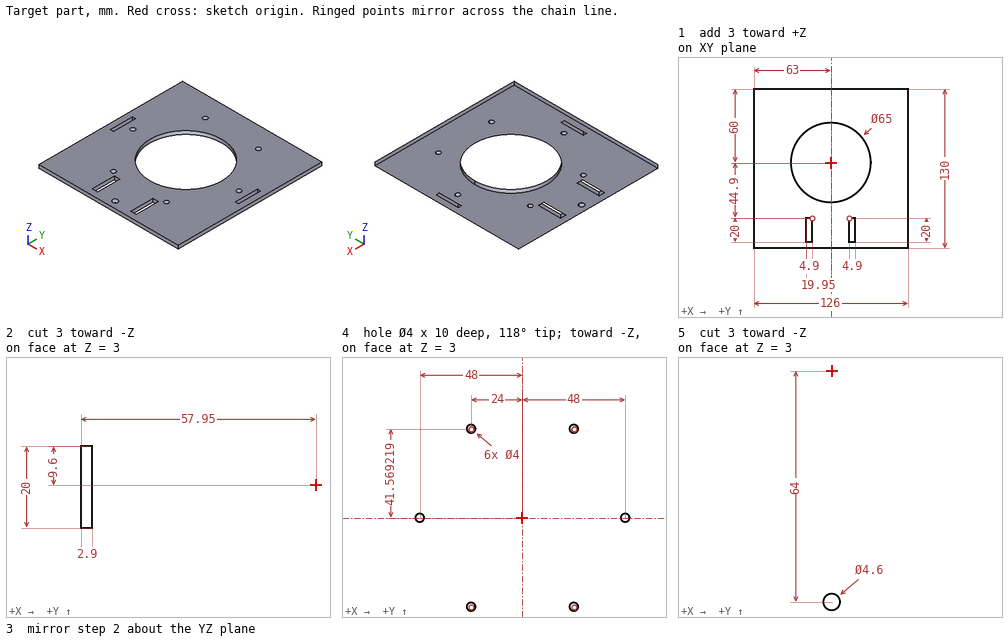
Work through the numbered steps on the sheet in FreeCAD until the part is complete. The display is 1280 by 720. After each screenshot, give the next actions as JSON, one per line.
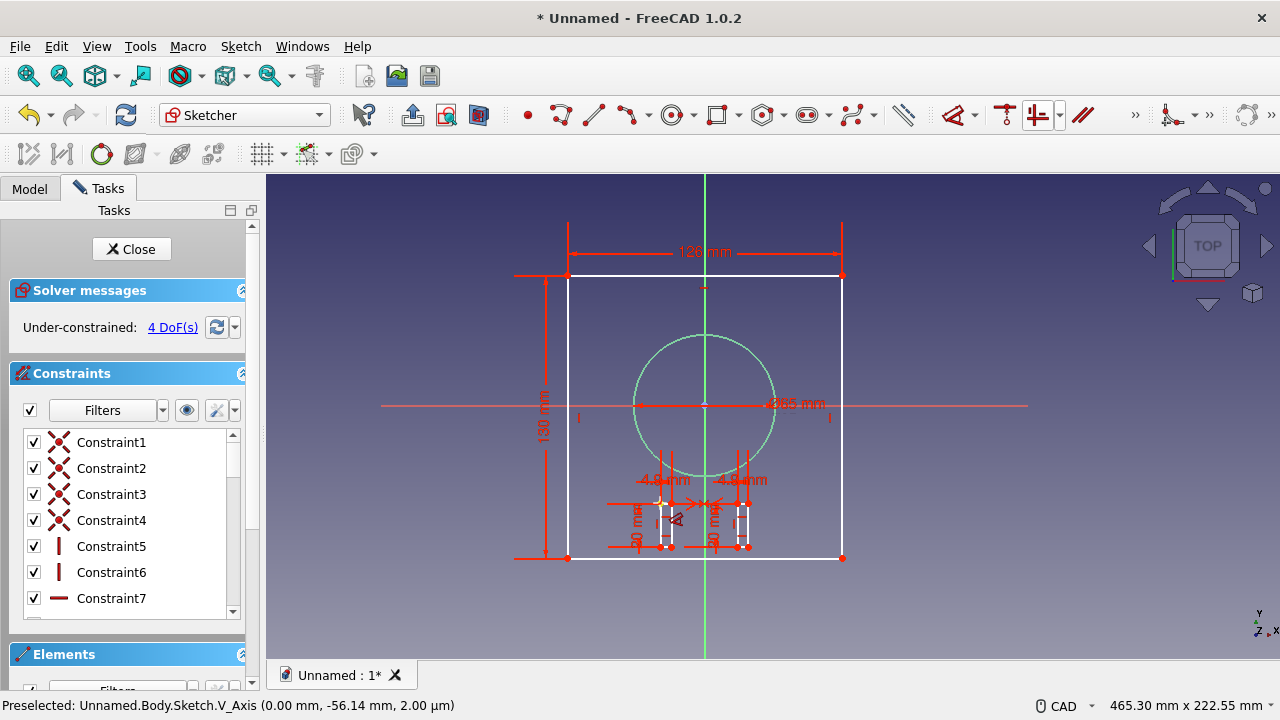
{"action": "left_click", "coordinate": [568, 276]}
{"action": "left_click", "coordinate": [636, 242]}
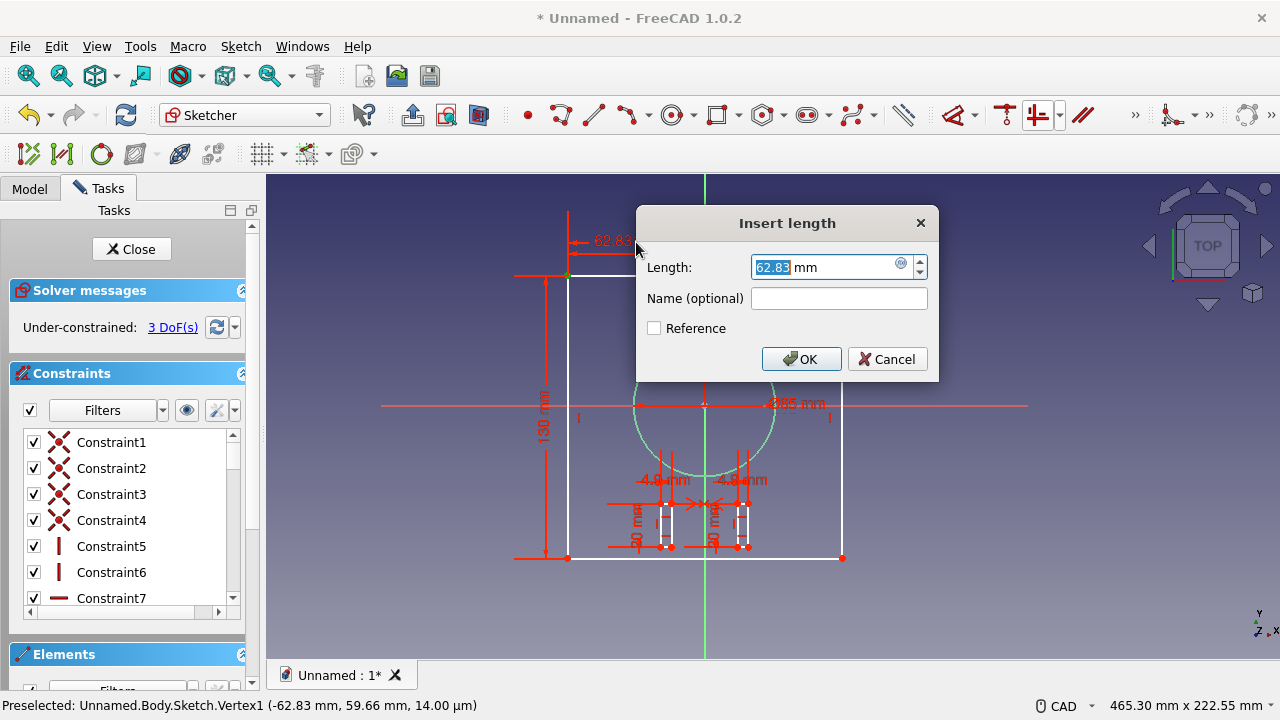
{"action": "type", "text": "63"}
{"action": "key", "text": "Return"}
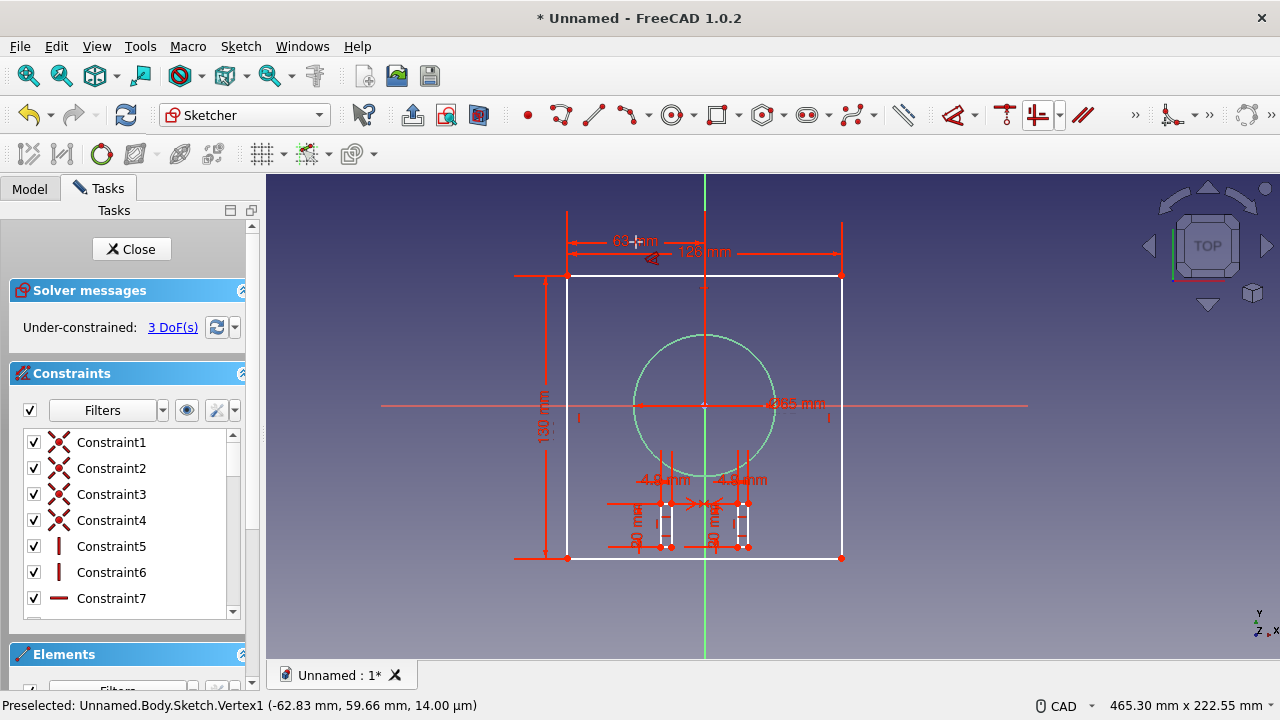
{"action": "left_click", "coordinate": [567, 276]}
{"action": "left_click", "coordinate": [533, 341]}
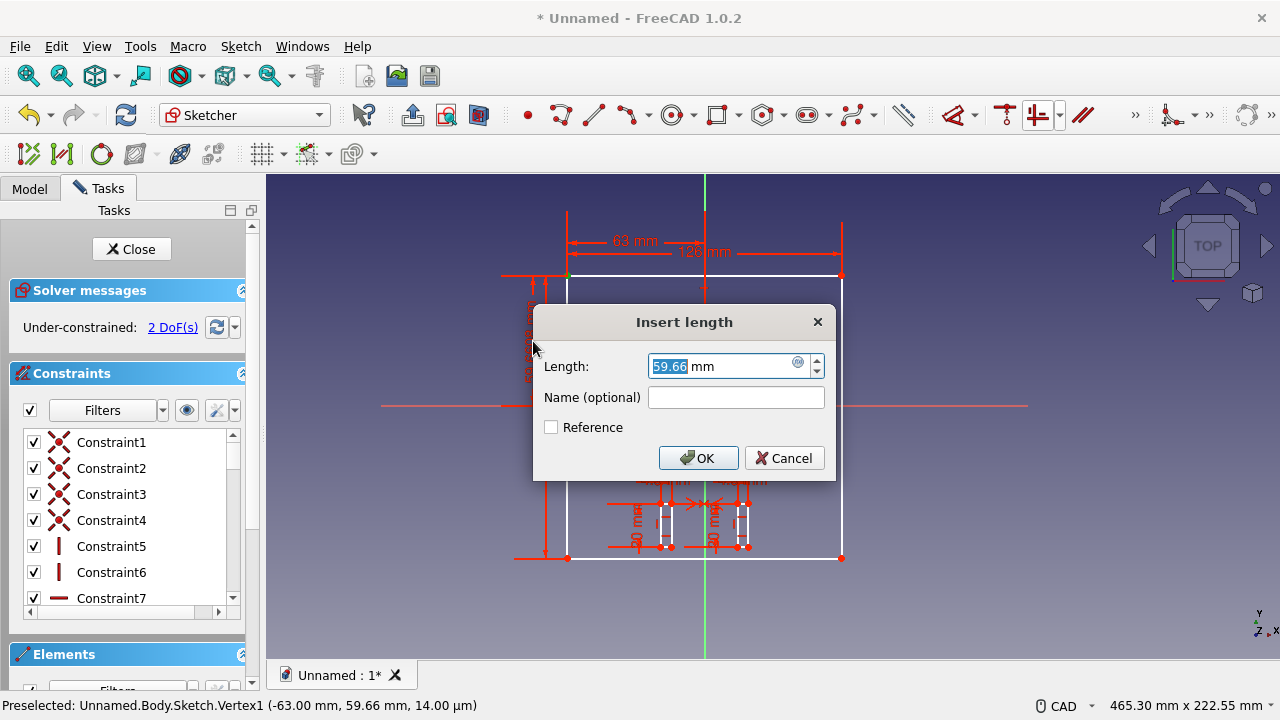
{"action": "type", "text": "60"}
{"action": "key", "text": "Return"}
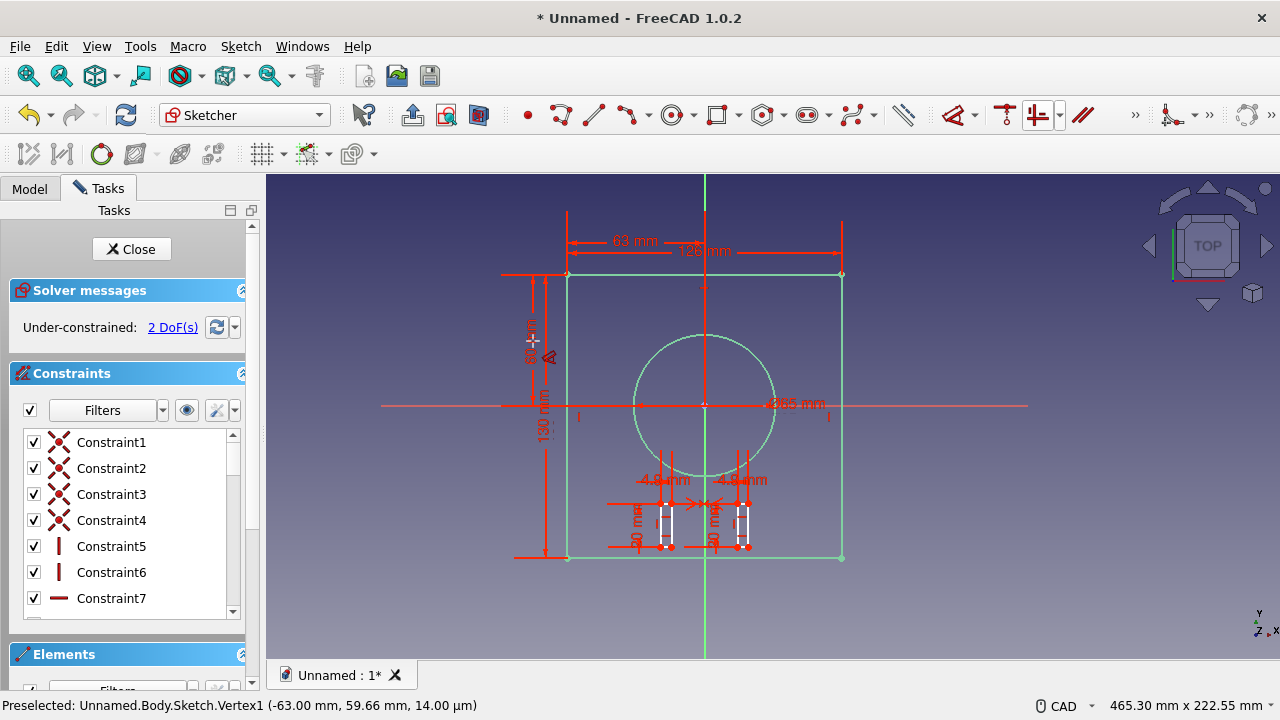
{"action": "left_click", "coordinate": [661, 504]}
{"action": "left_click", "coordinate": [627, 455]}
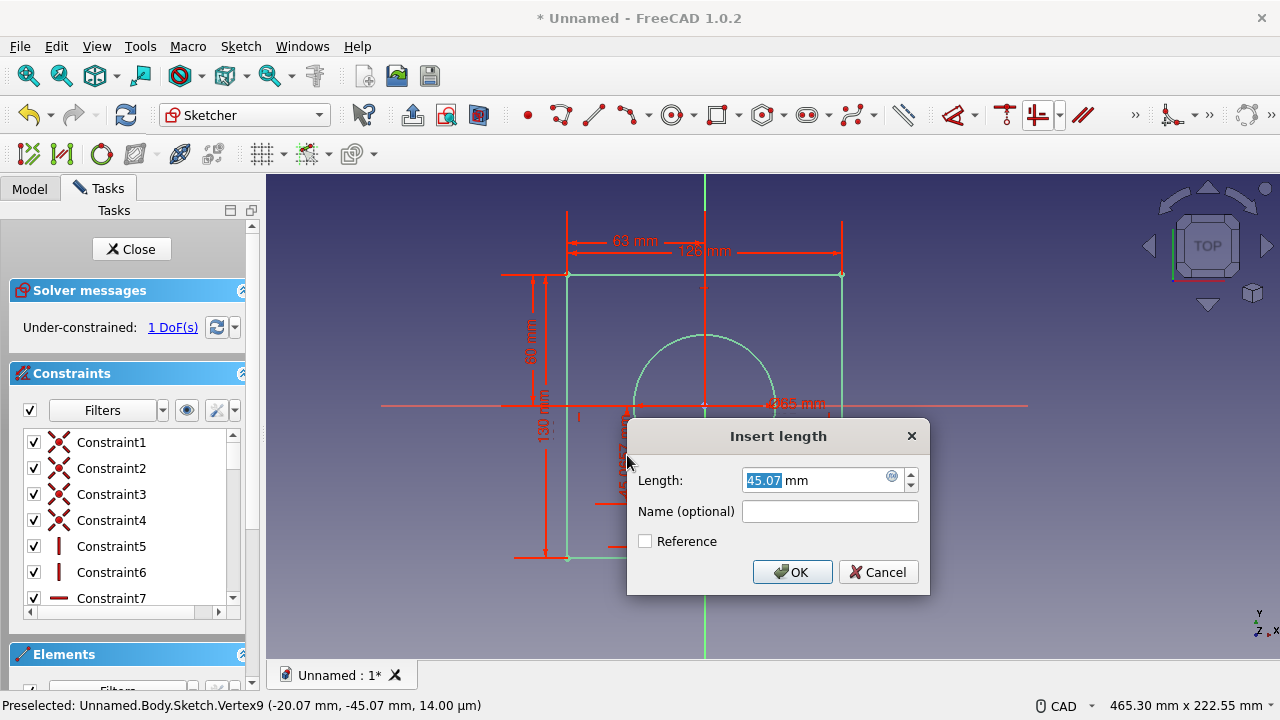
{"action": "type", "text": "44.9"}
{"action": "key", "text": "Return"}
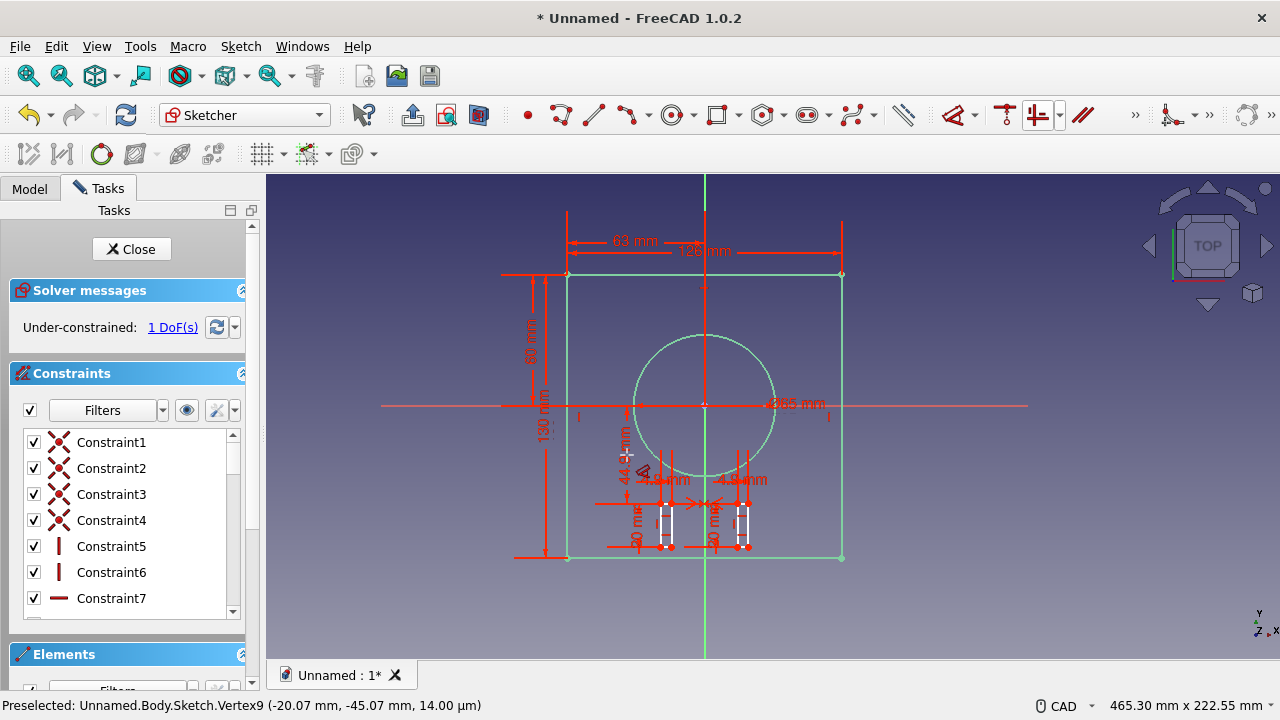
{"action": "left_click", "coordinate": [661, 504]}
{"action": "left_click", "coordinate": [683, 372]}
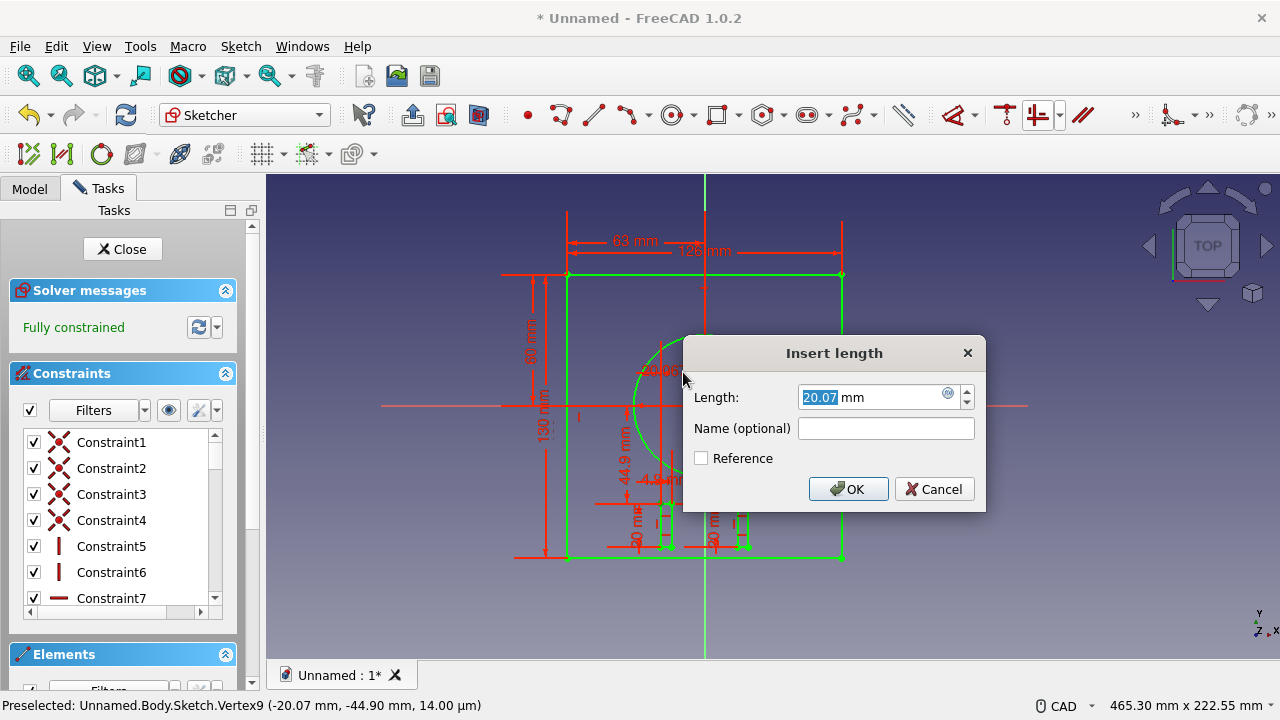
{"action": "type", "text": "19.95"}
{"action": "key", "text": "Return"}
{"action": "key", "text": "Escape"}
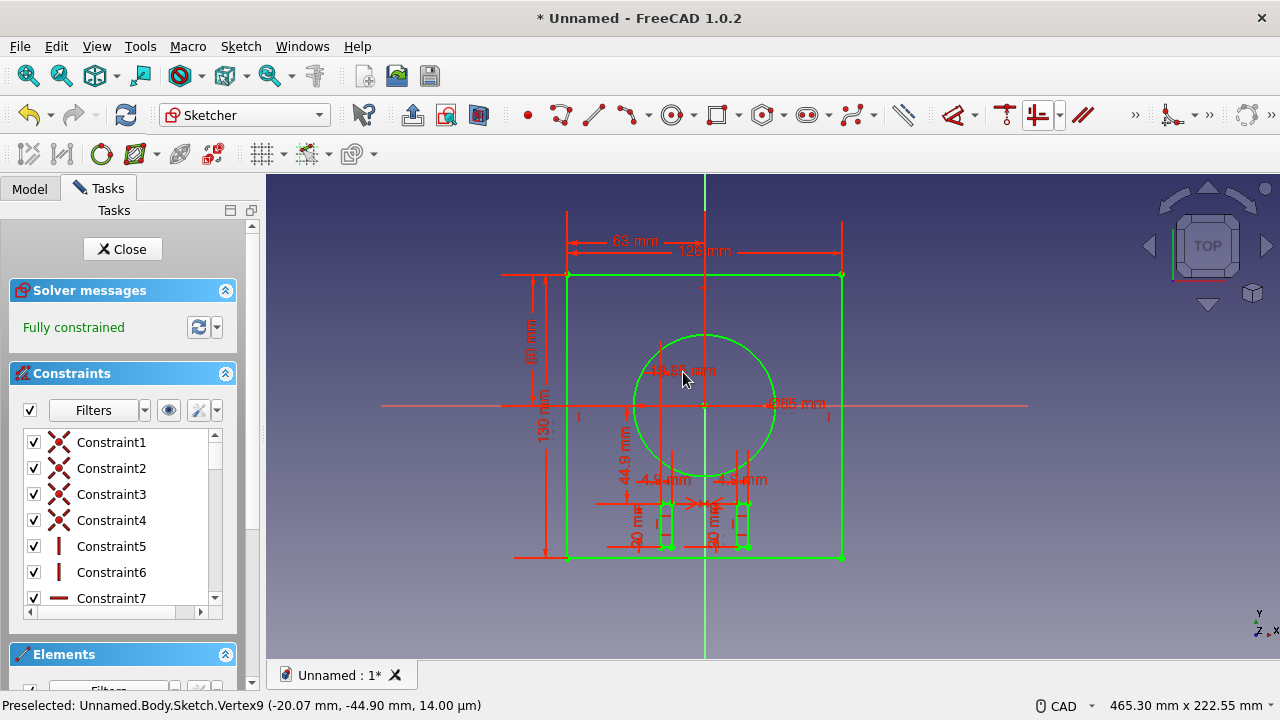
{"action": "left_click", "coordinate": [123, 249]}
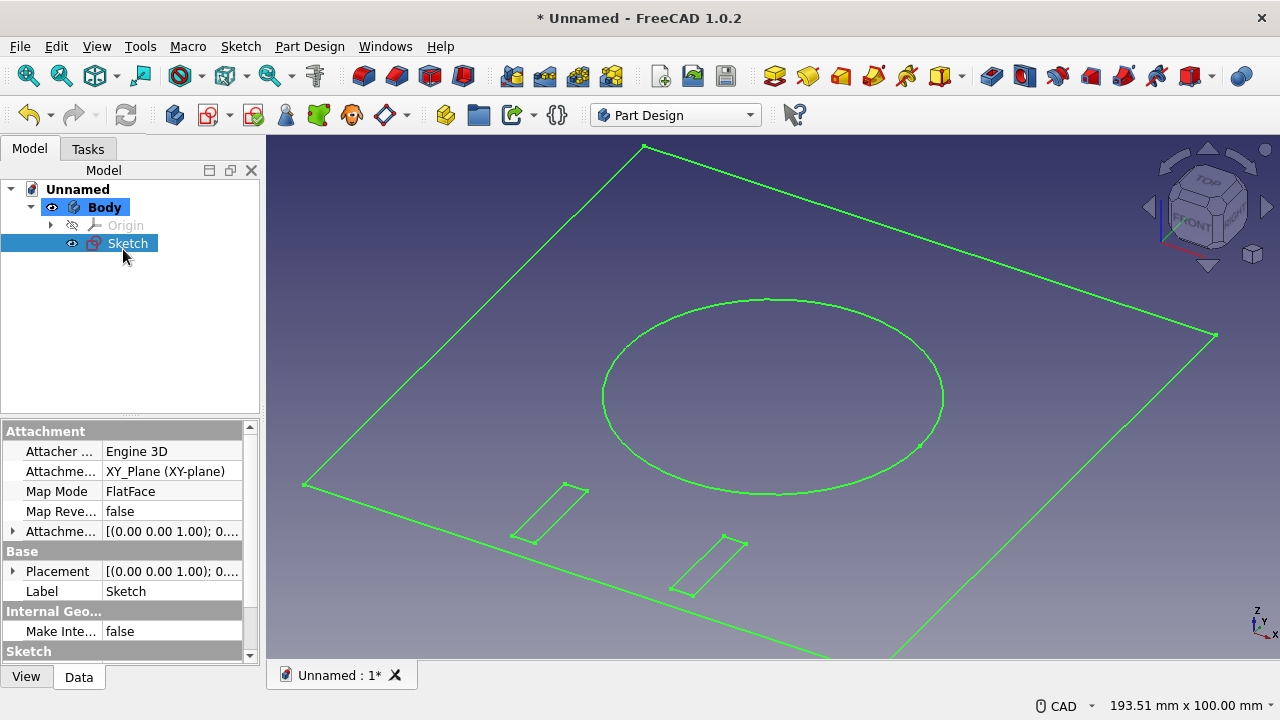
{"action": "left_click", "coordinate": [775, 76]}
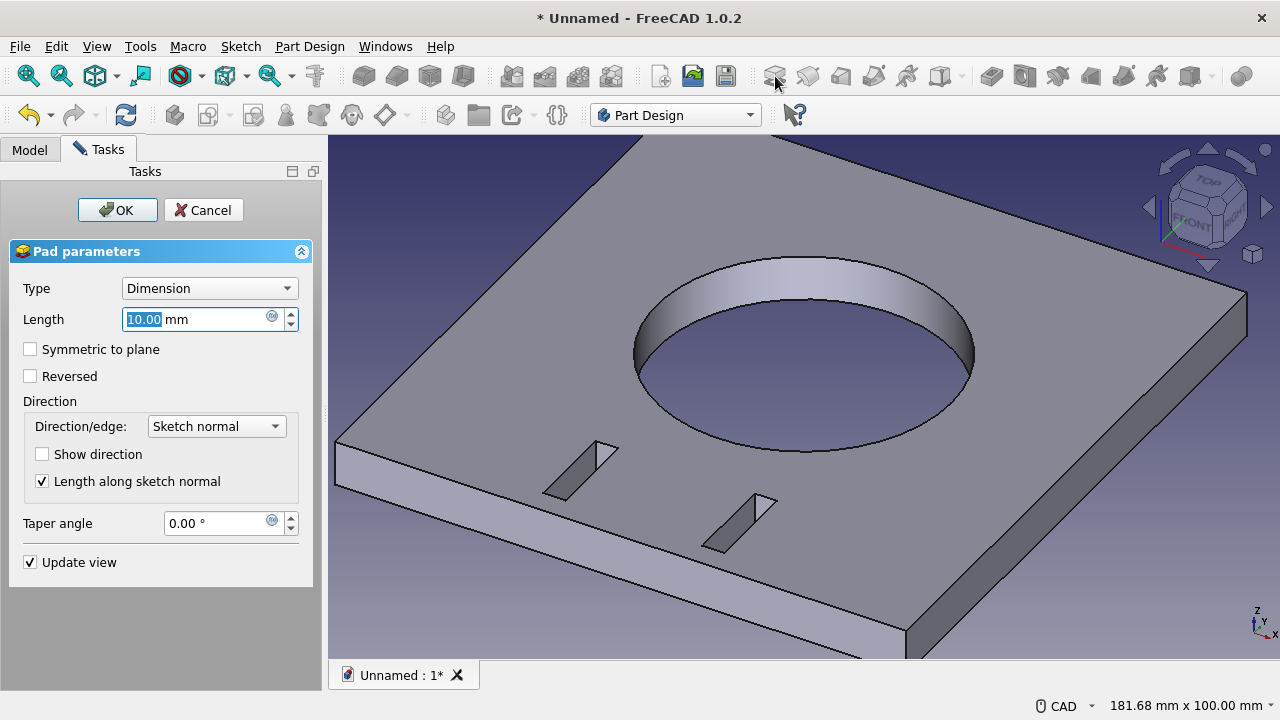
{"action": "type", "text": "3"}
{"action": "key", "text": "Tab"}